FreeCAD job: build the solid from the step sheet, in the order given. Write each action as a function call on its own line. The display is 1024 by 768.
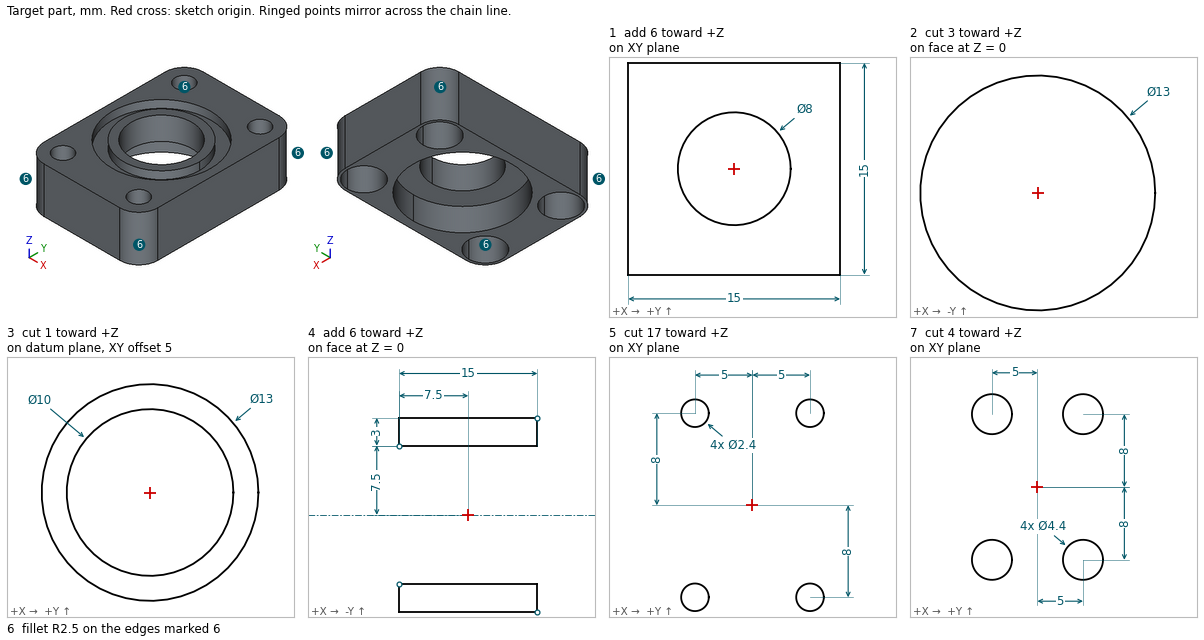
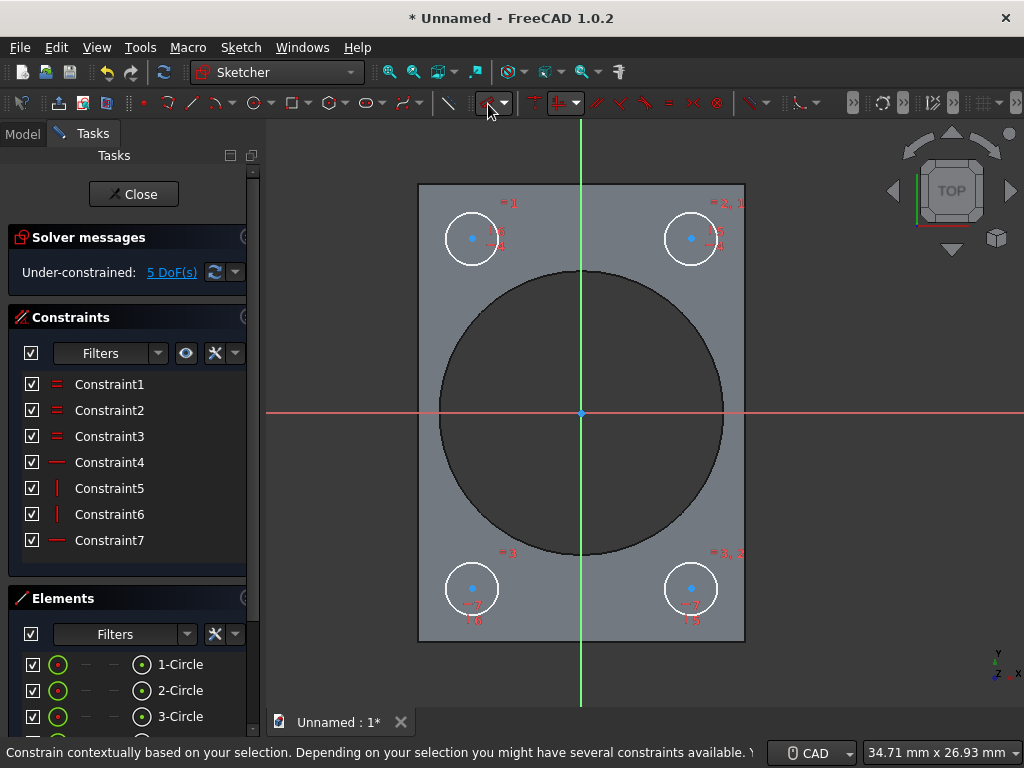
click(490, 220)
click(512, 197)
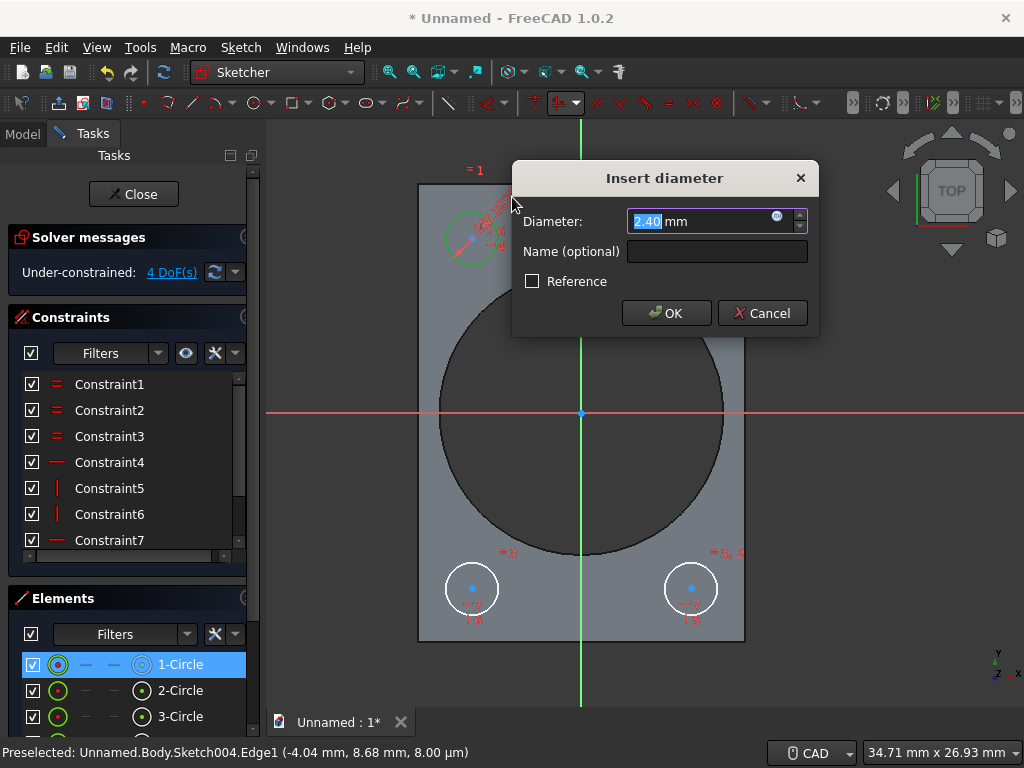
text(2.4)
key(Return)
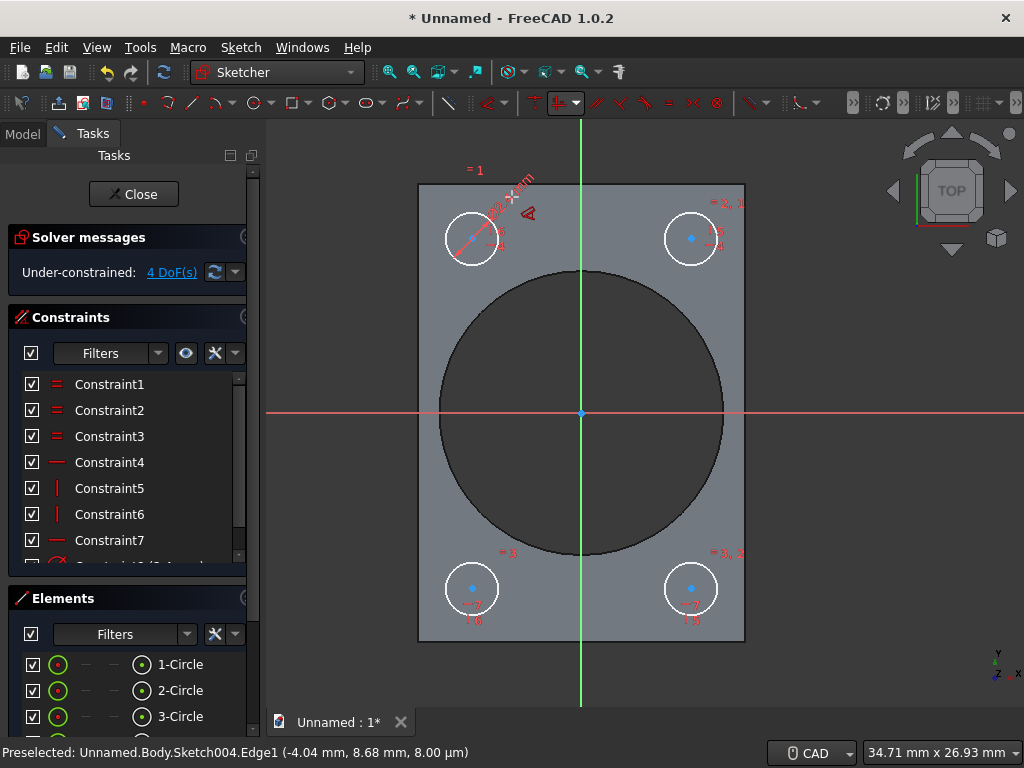
click(472, 239)
click(527, 447)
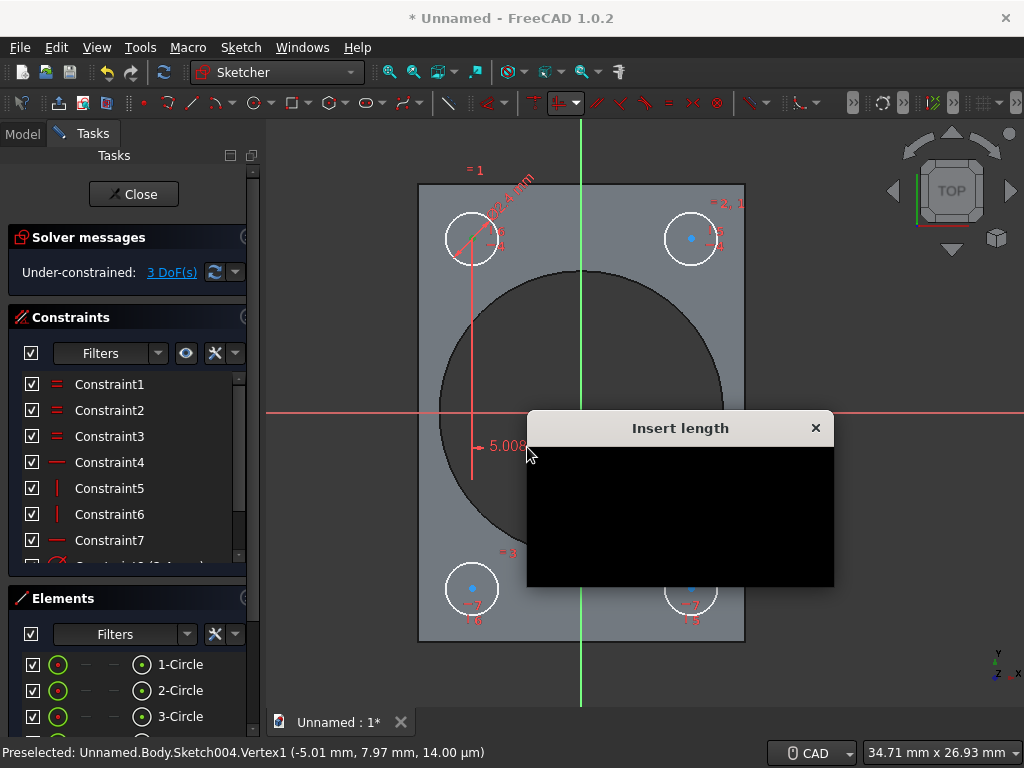
text(5)
key(Return)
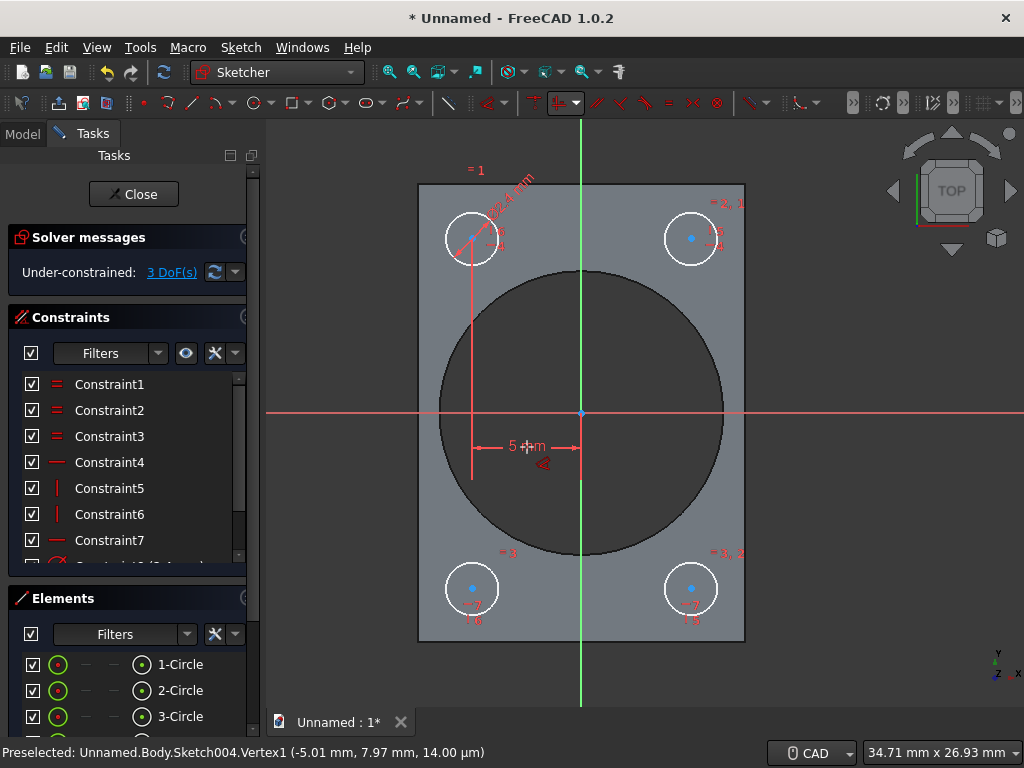
click(472, 239)
click(438, 326)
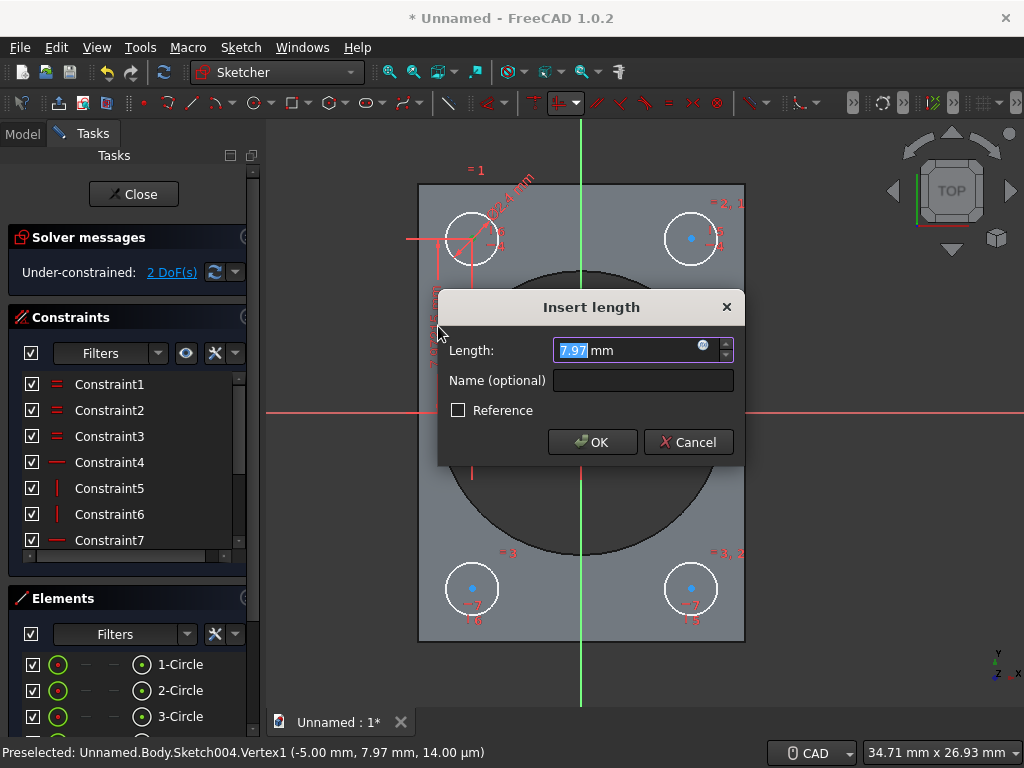
text(8)
key(Return)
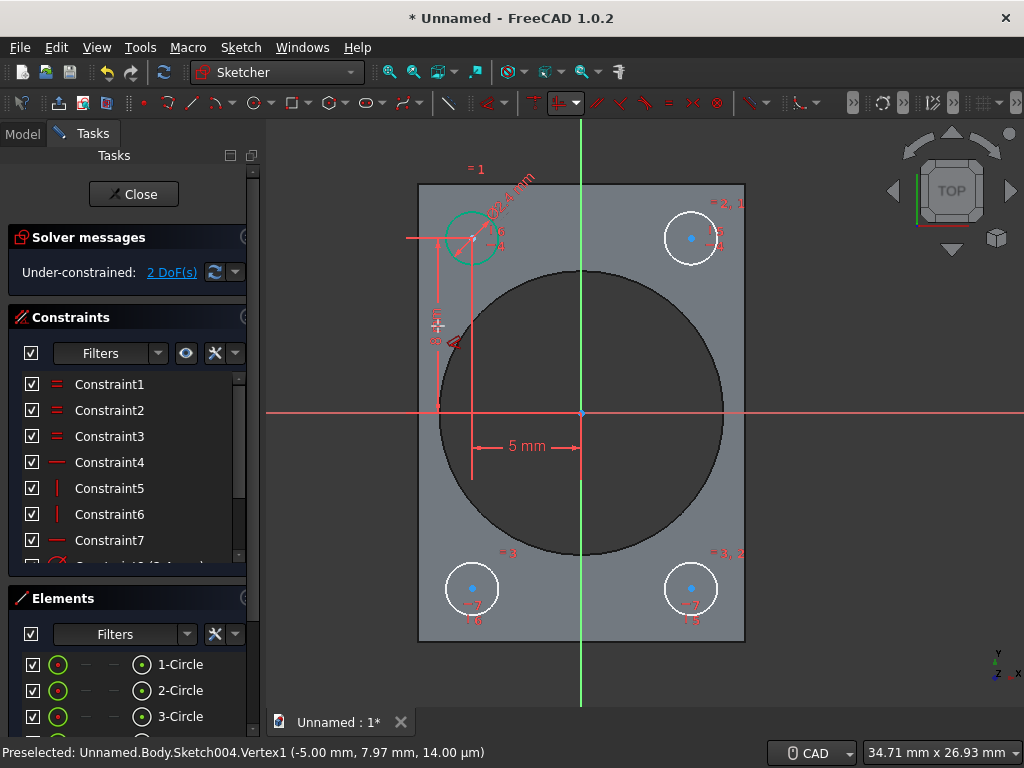
click(691, 238)
click(636, 204)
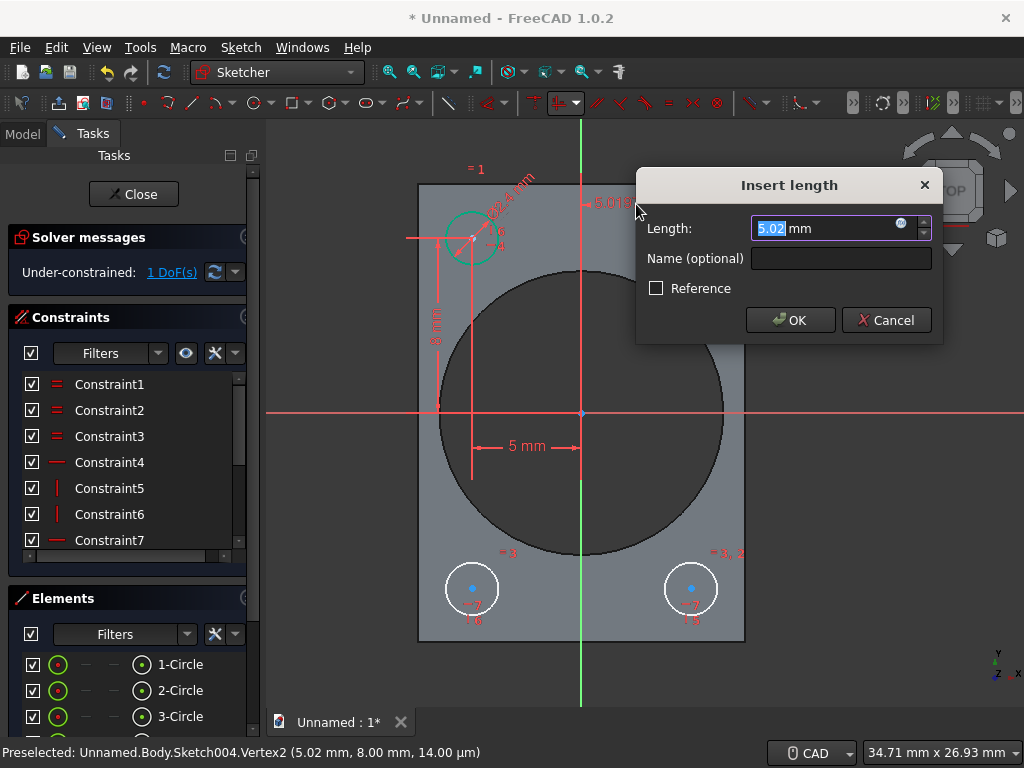
text(5)
key(Return)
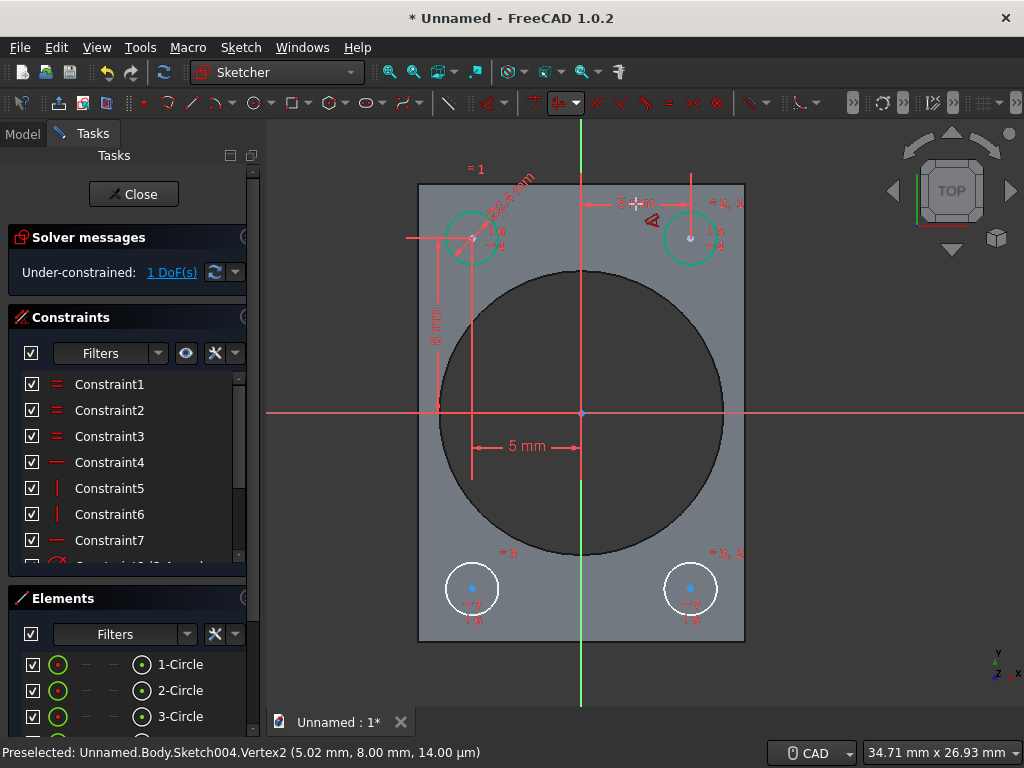
click(691, 589)
click(725, 501)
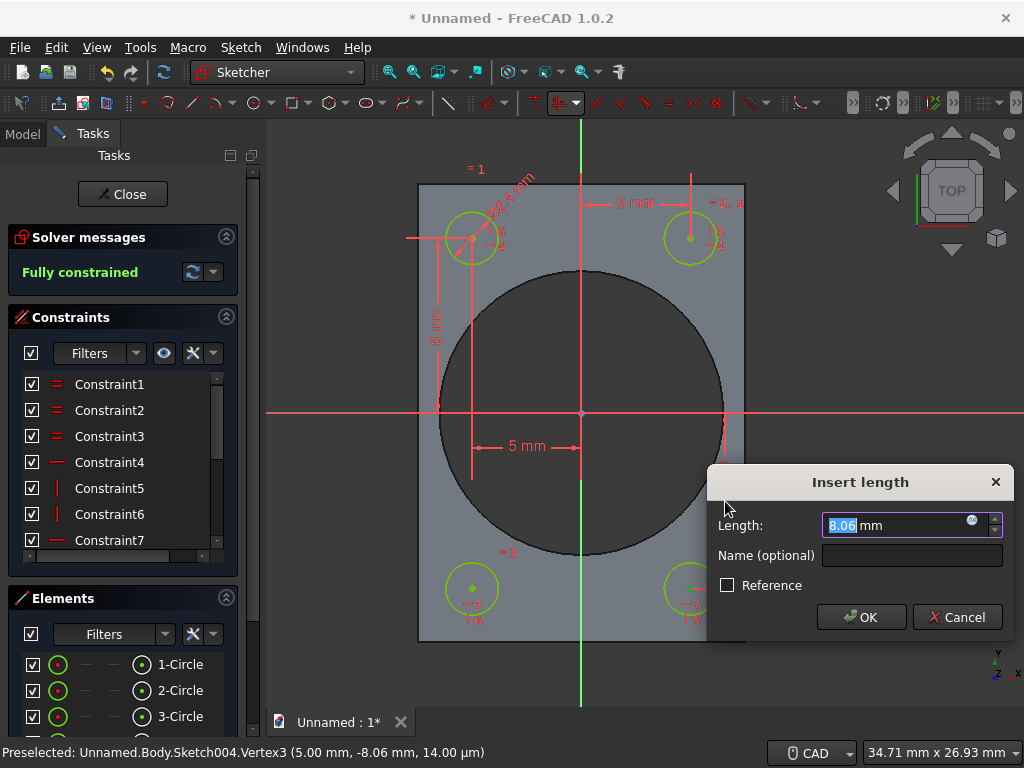
text(8)
key(Return)
key(Escape)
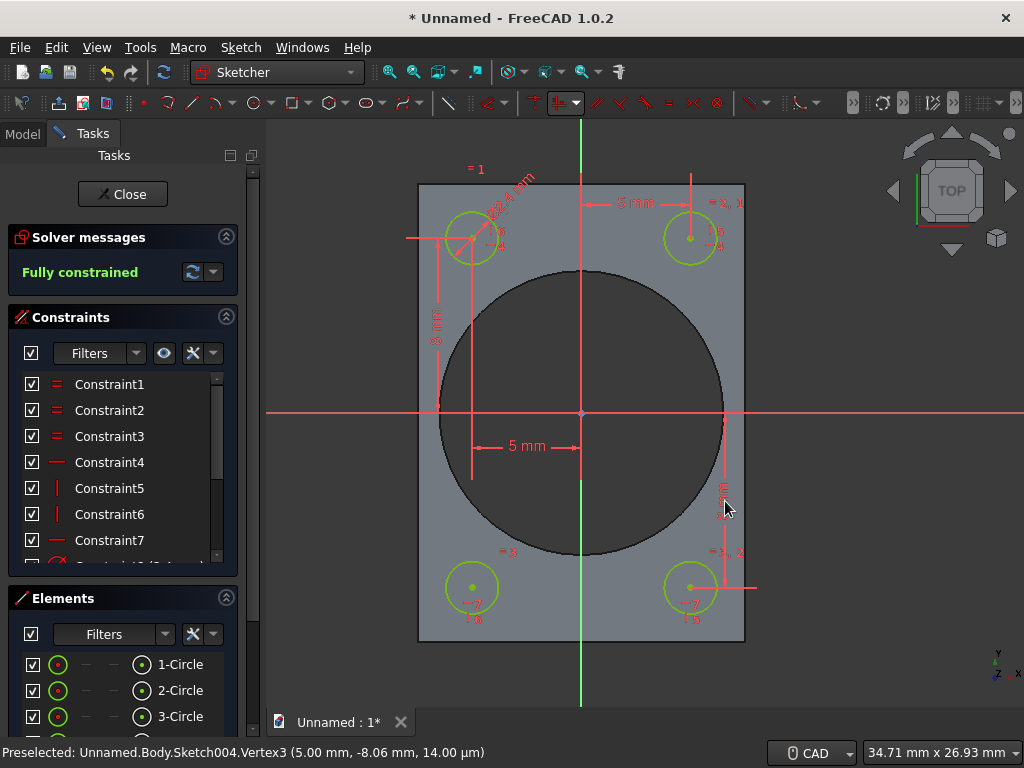
click(123, 194)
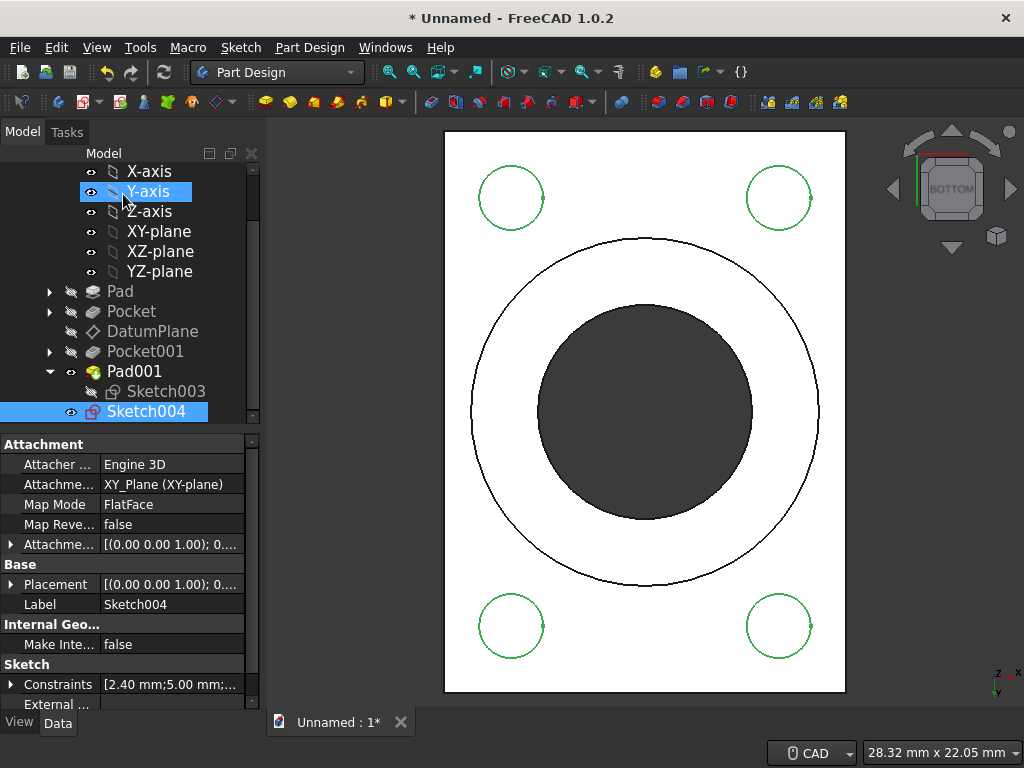
click(432, 102)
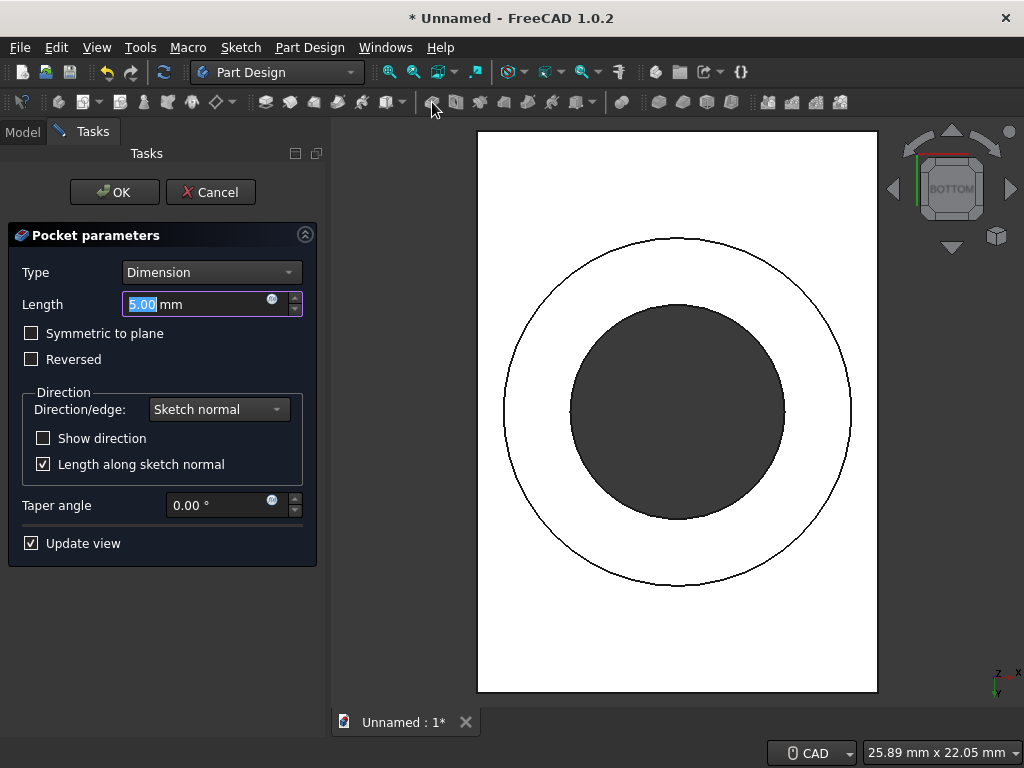
text(17)
key(Tab)